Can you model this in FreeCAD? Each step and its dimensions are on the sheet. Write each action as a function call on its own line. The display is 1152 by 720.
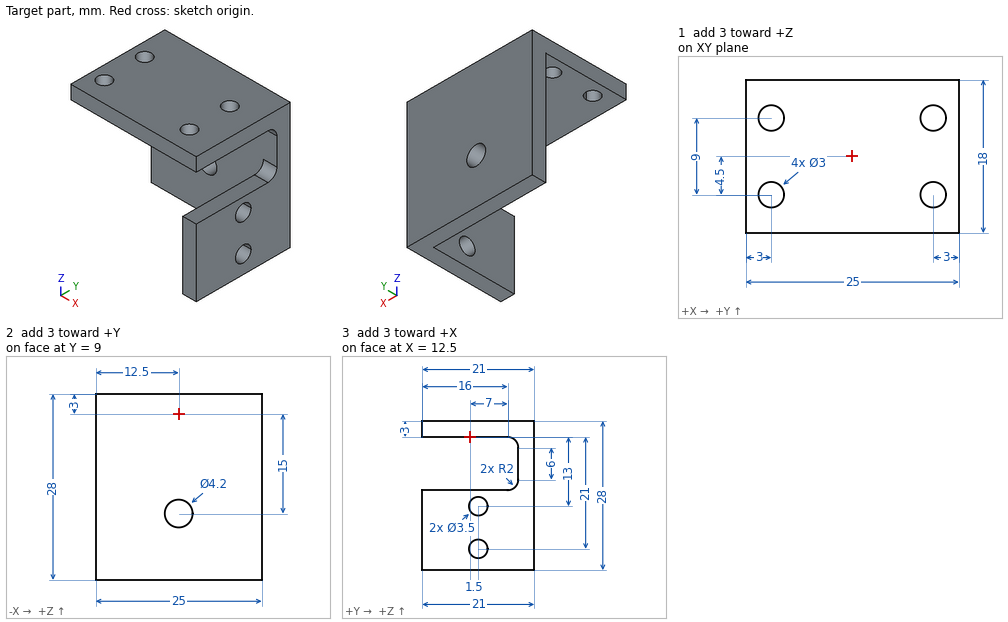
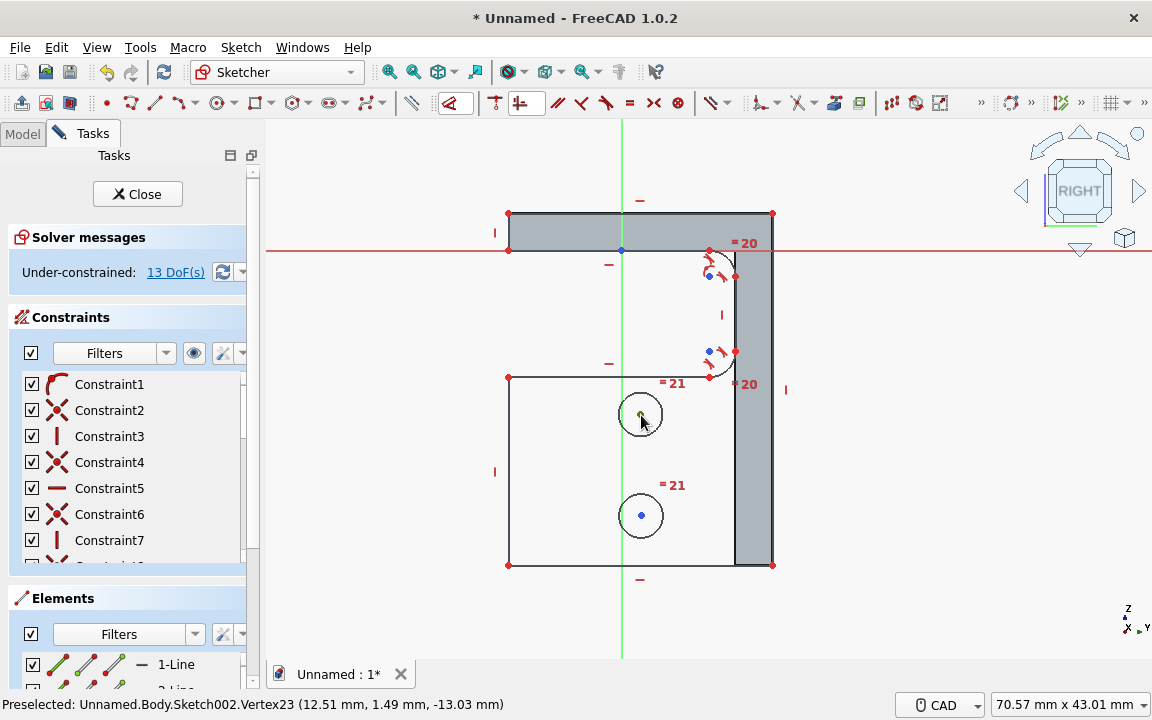
click(641, 516)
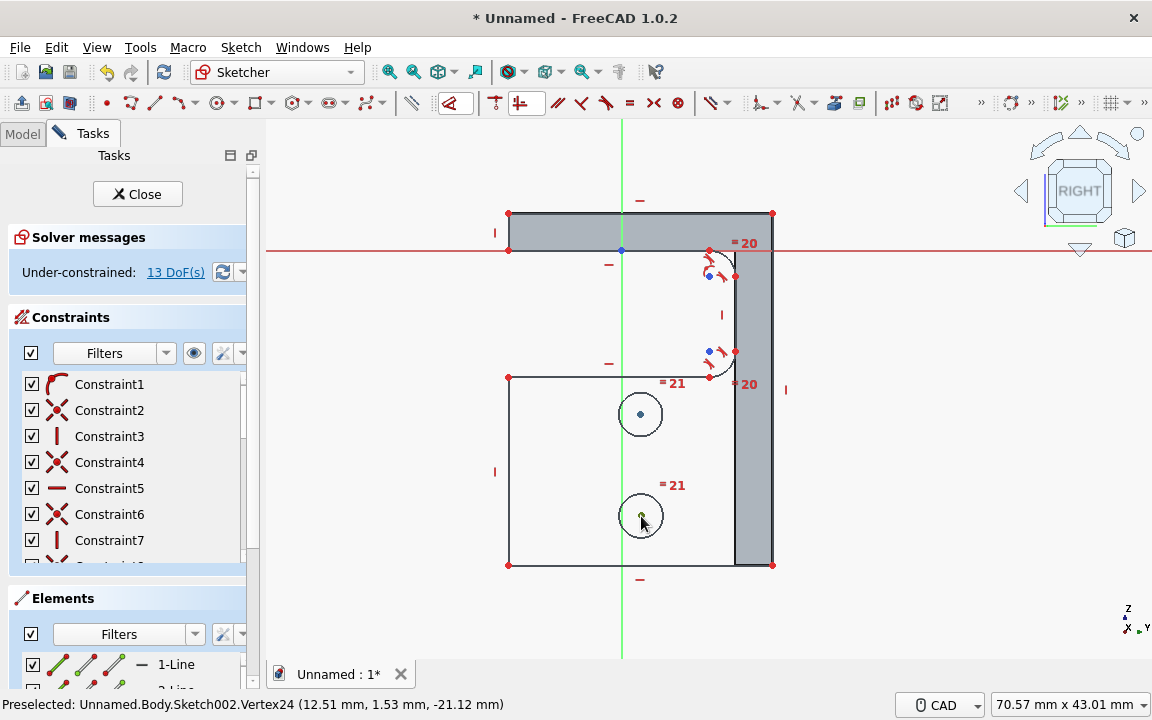
key(v)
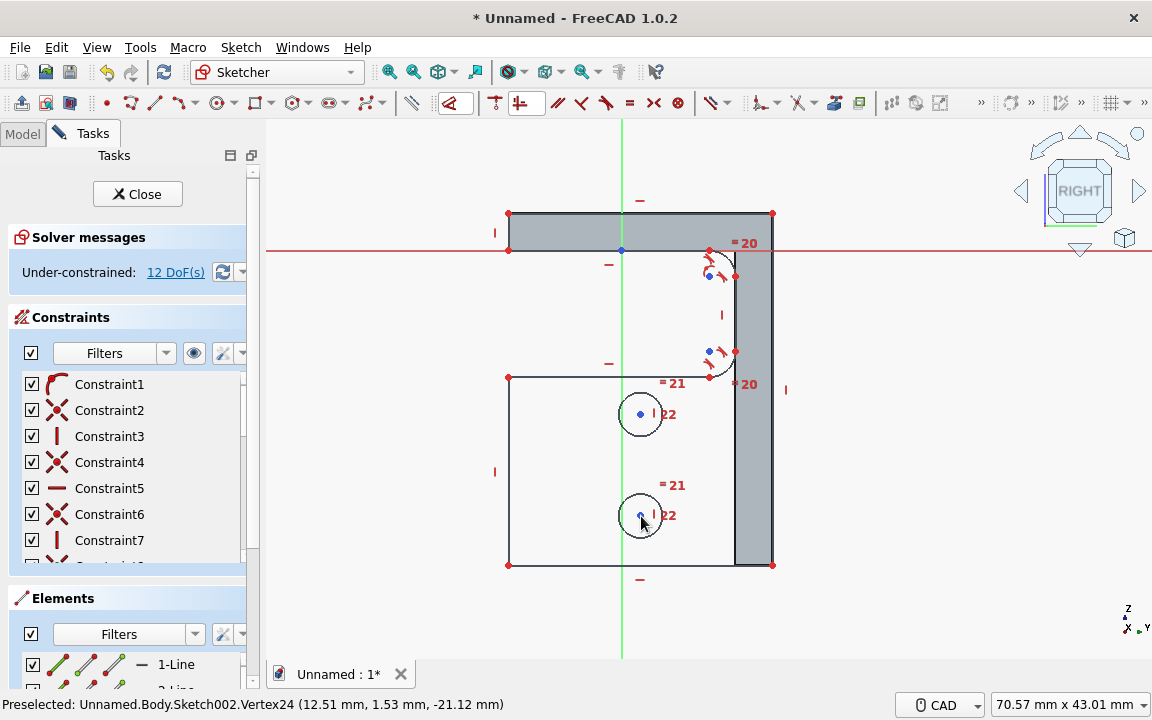
scroll(721, 374, up, 3)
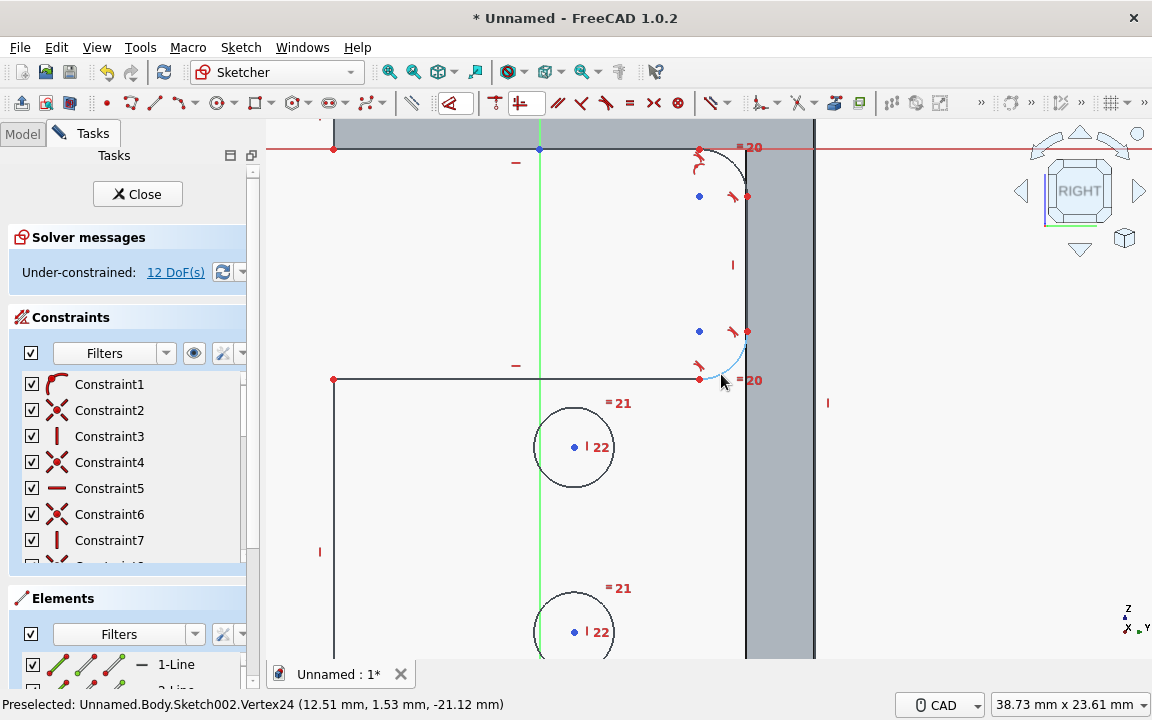
click(721, 374)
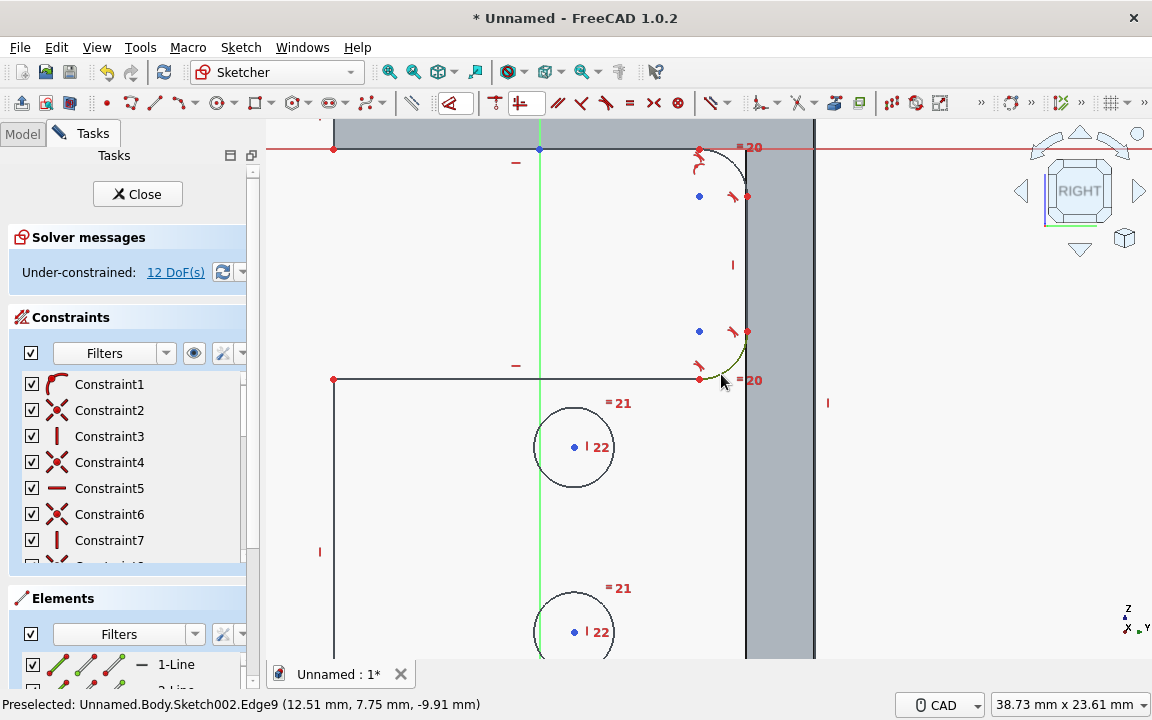
key(k)
key(r)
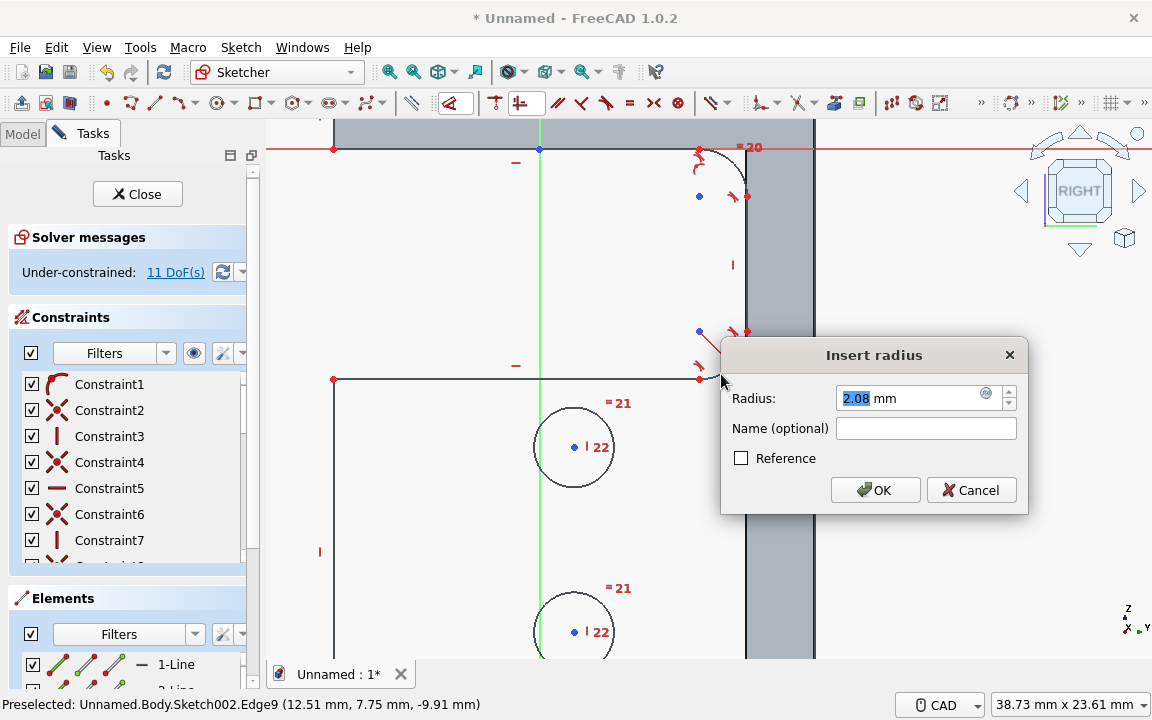
text(2)
key(Return)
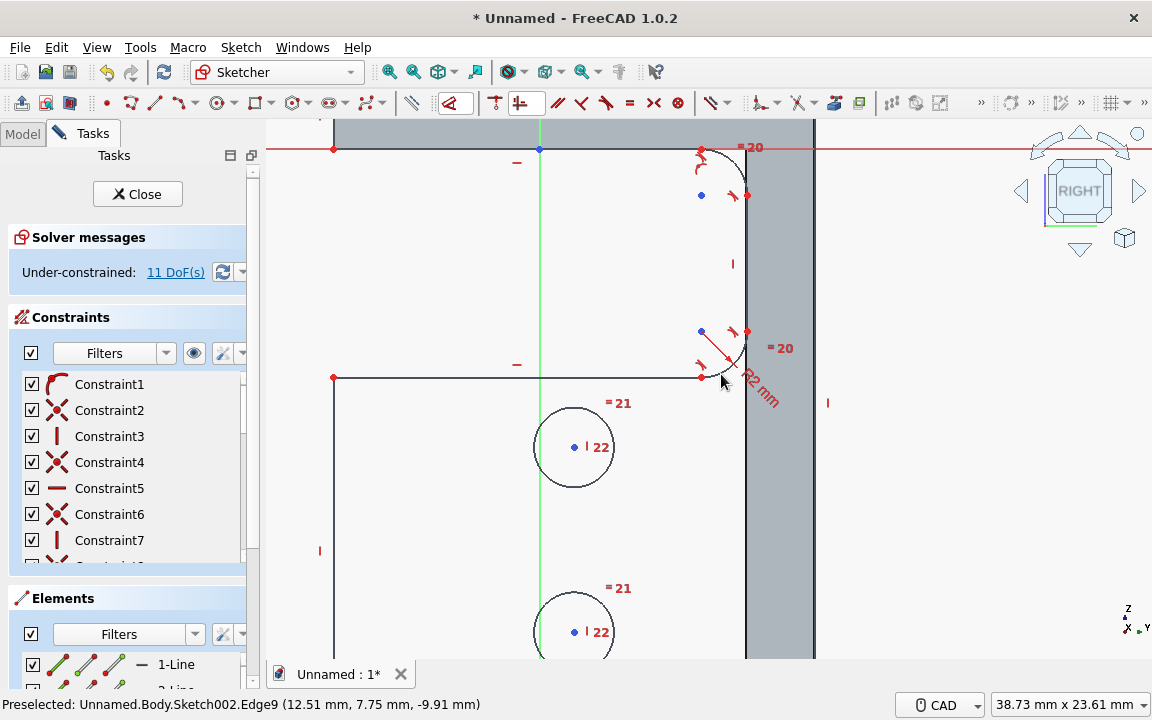
click(602, 419)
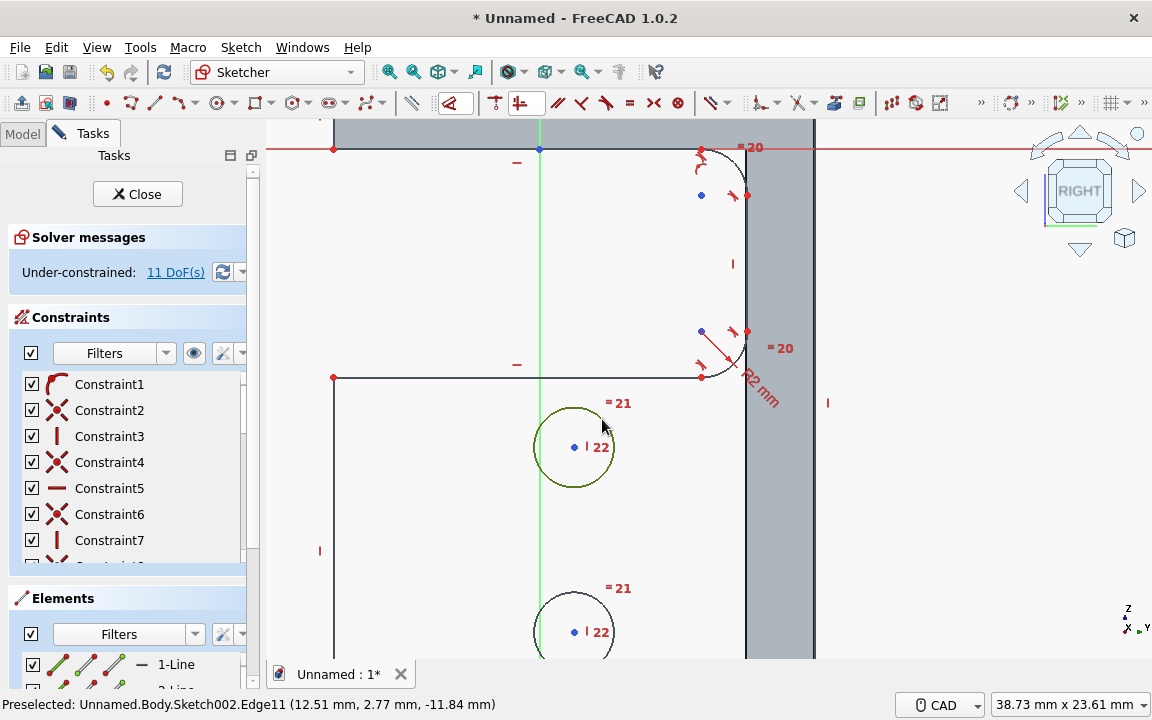
key(k)
key(o)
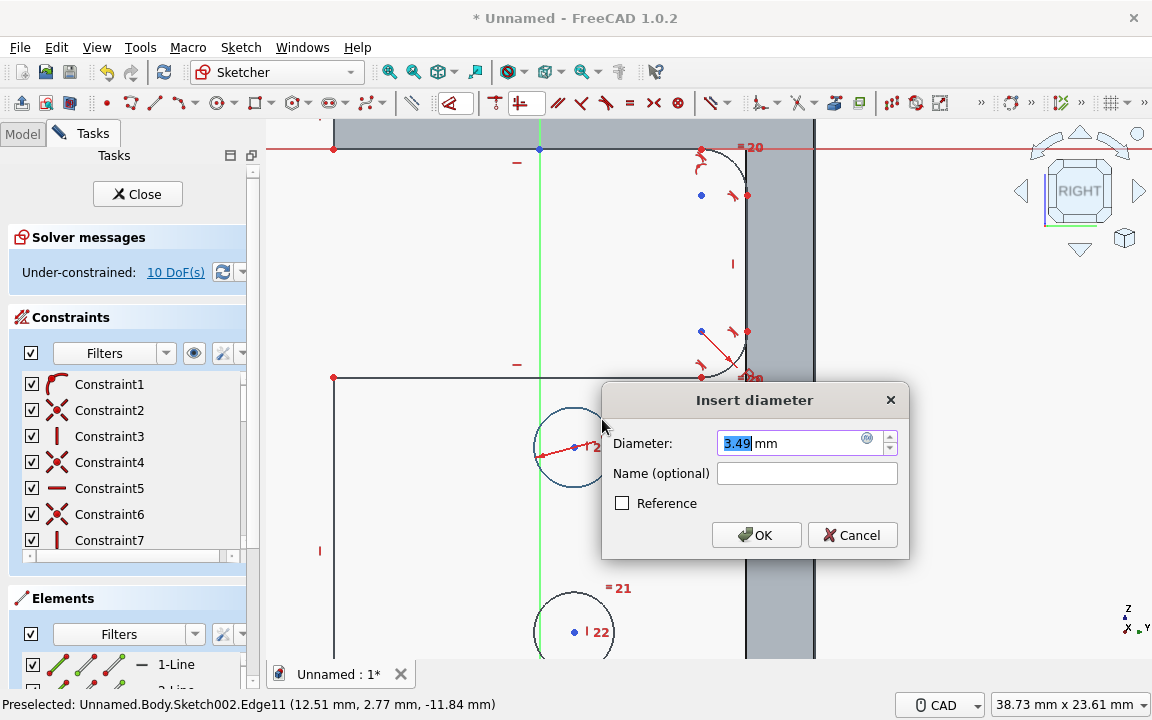
text(3.5)
key(Return)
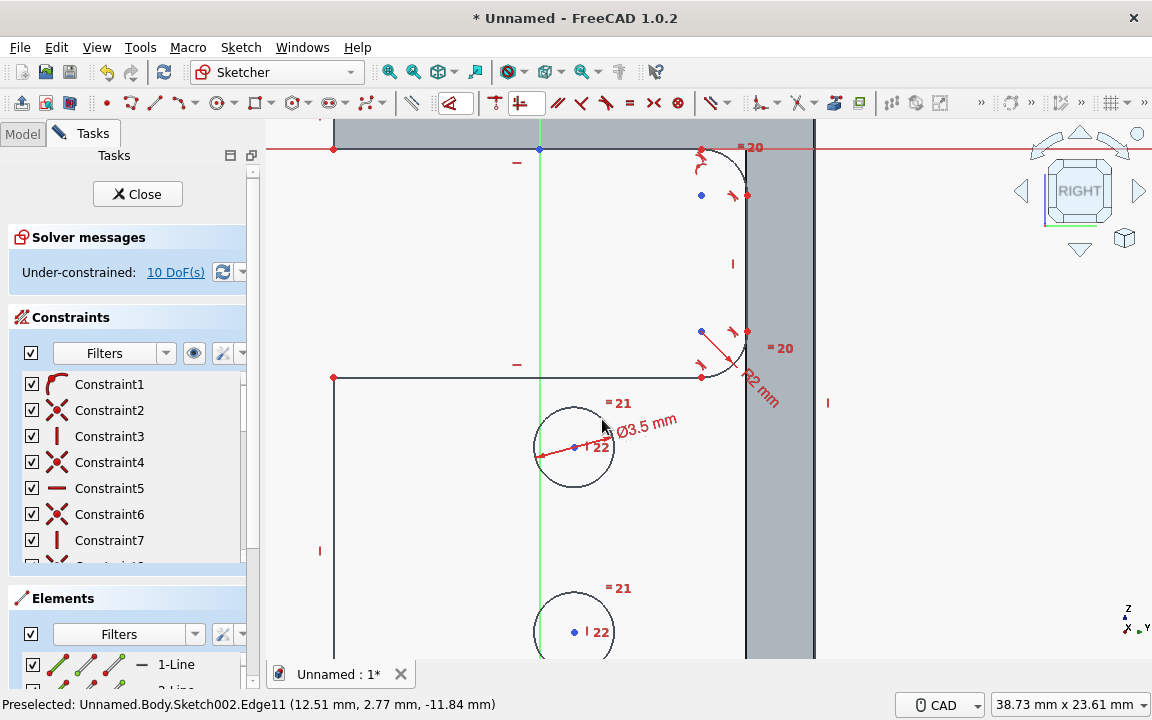
scroll(721, 374, down, 3)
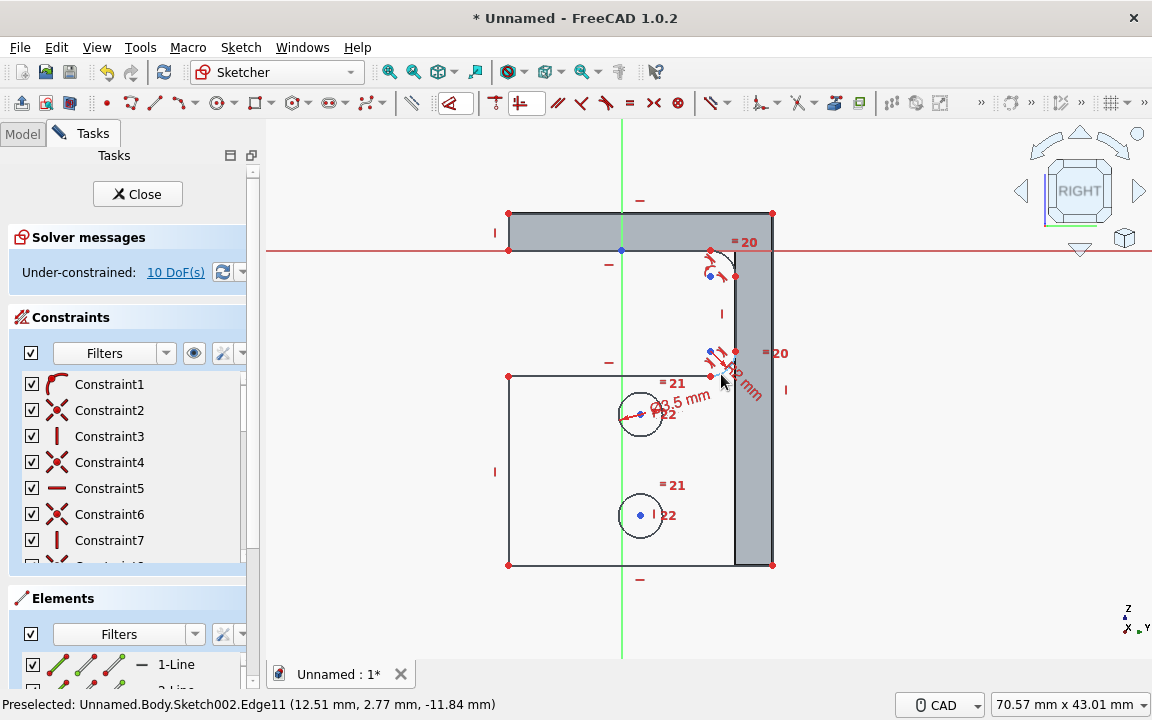
scroll(509, 240, up, 2)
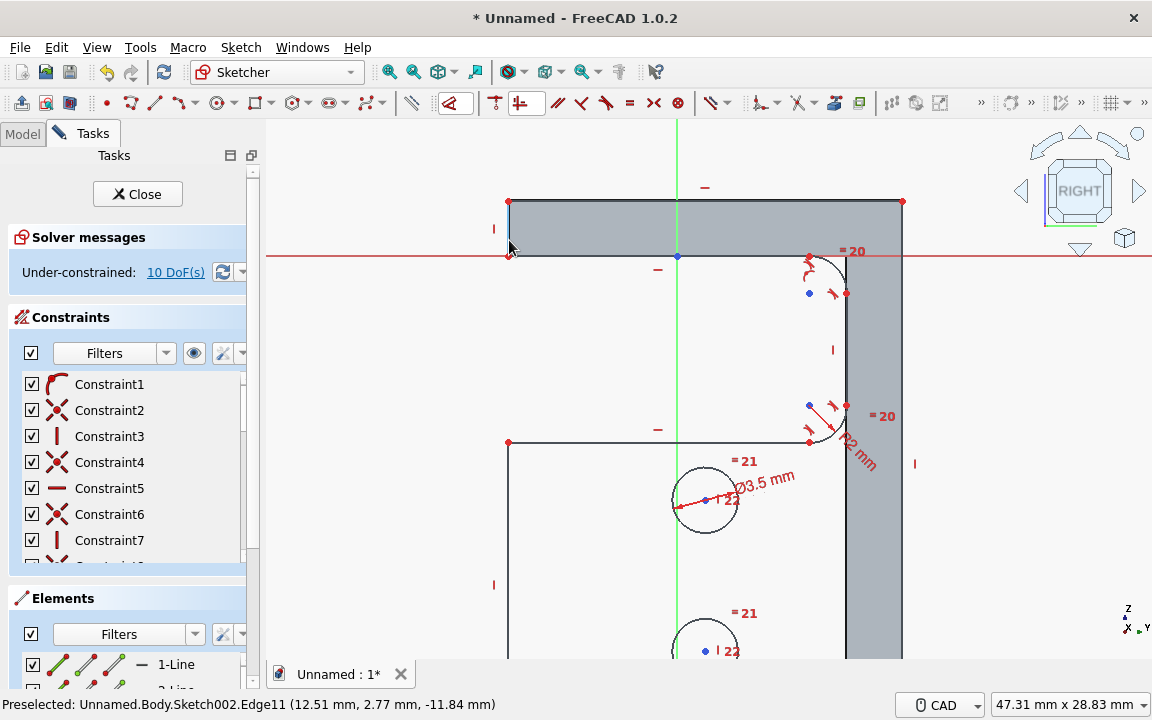
click(508, 240)